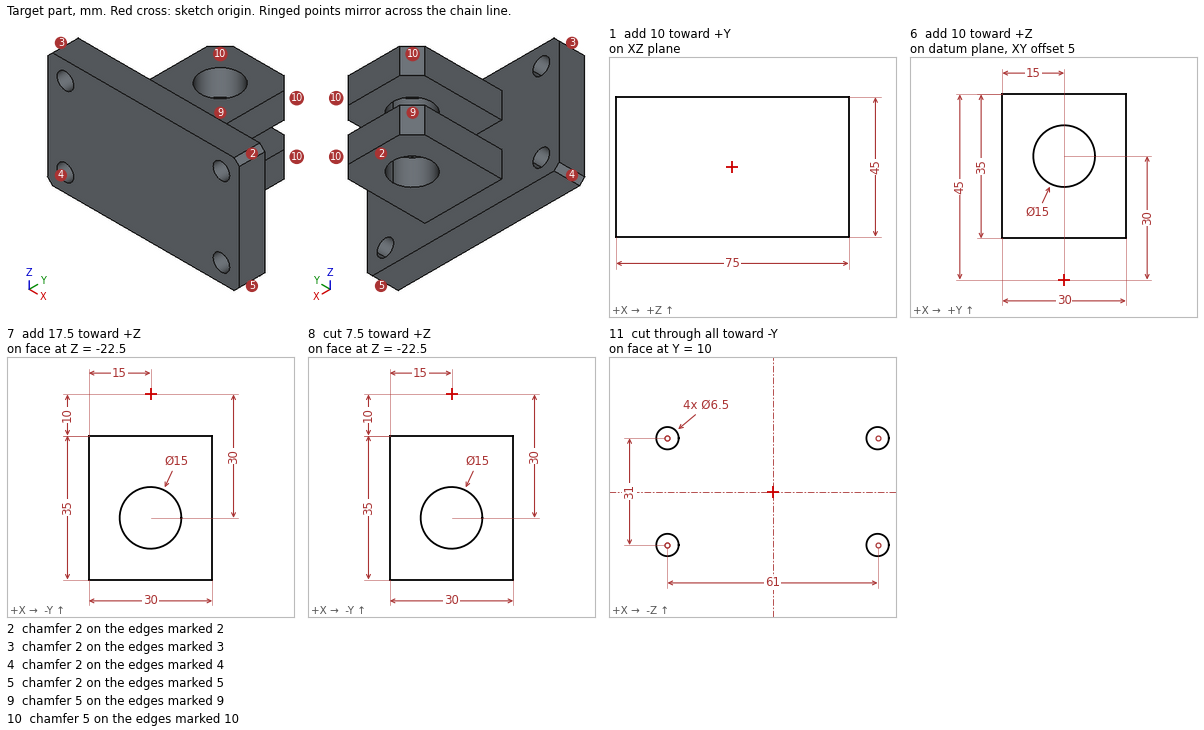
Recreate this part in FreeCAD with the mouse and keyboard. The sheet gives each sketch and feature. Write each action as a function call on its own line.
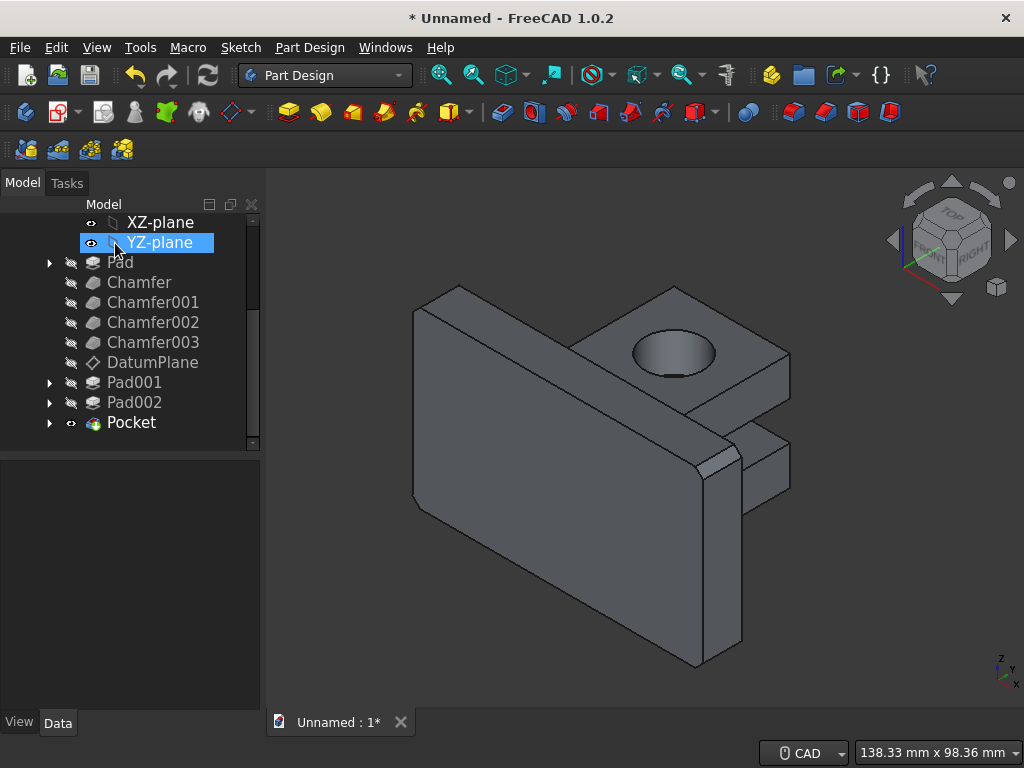
key(2)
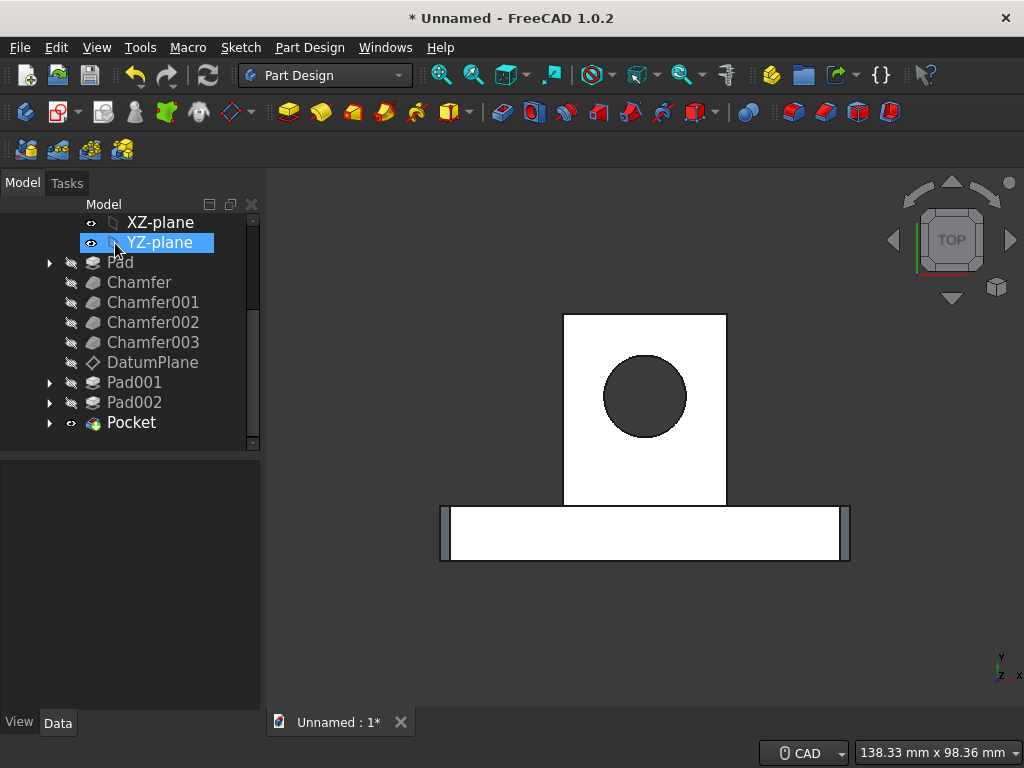
key(1)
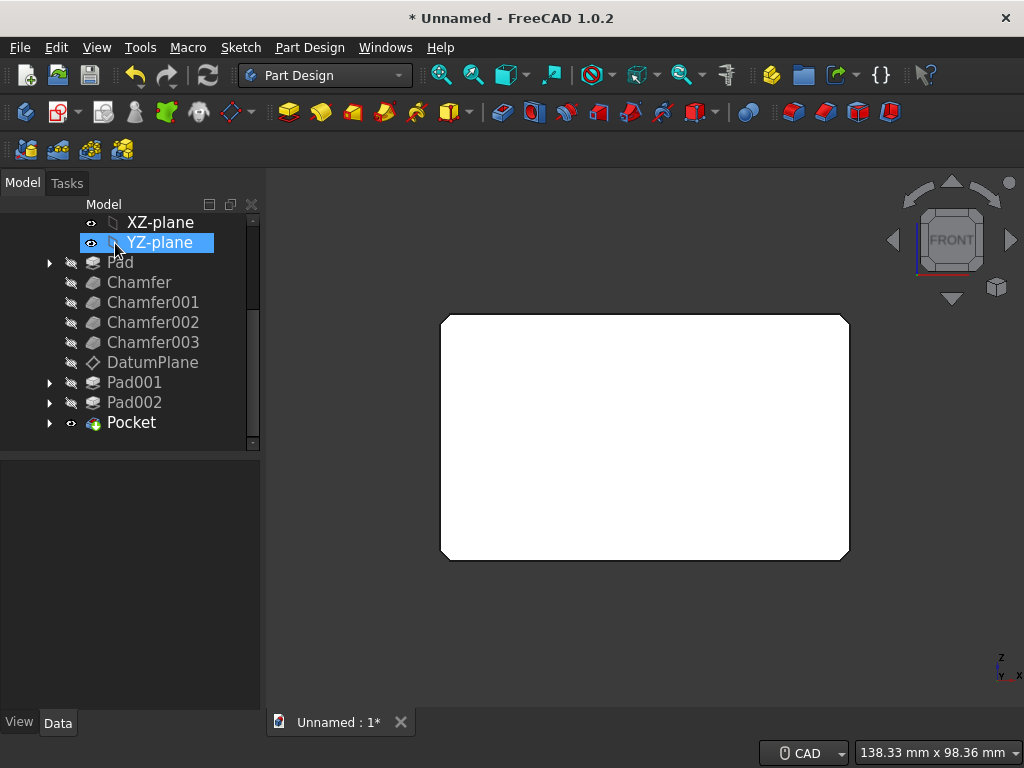
key(3)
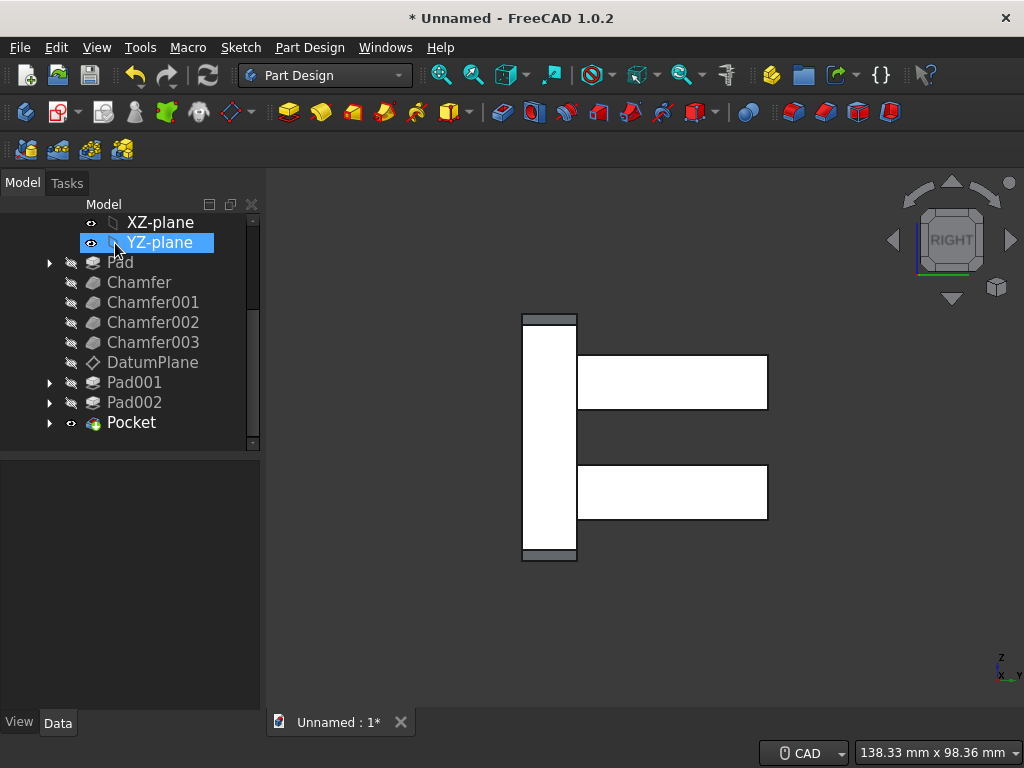
key(5)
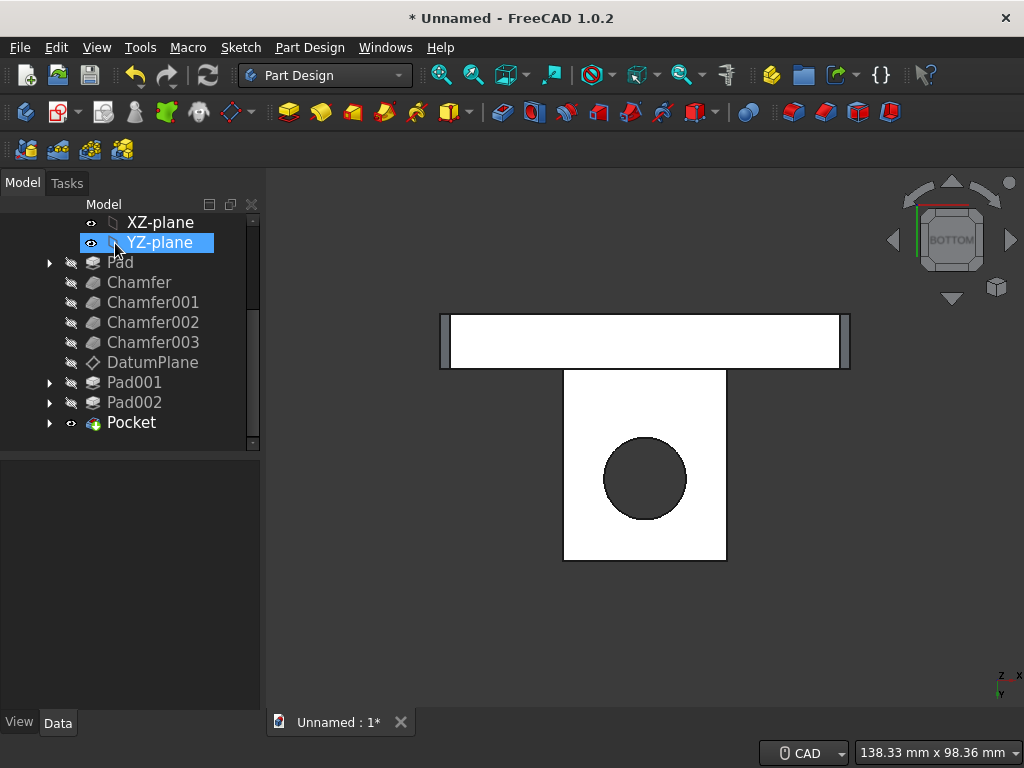
key(4)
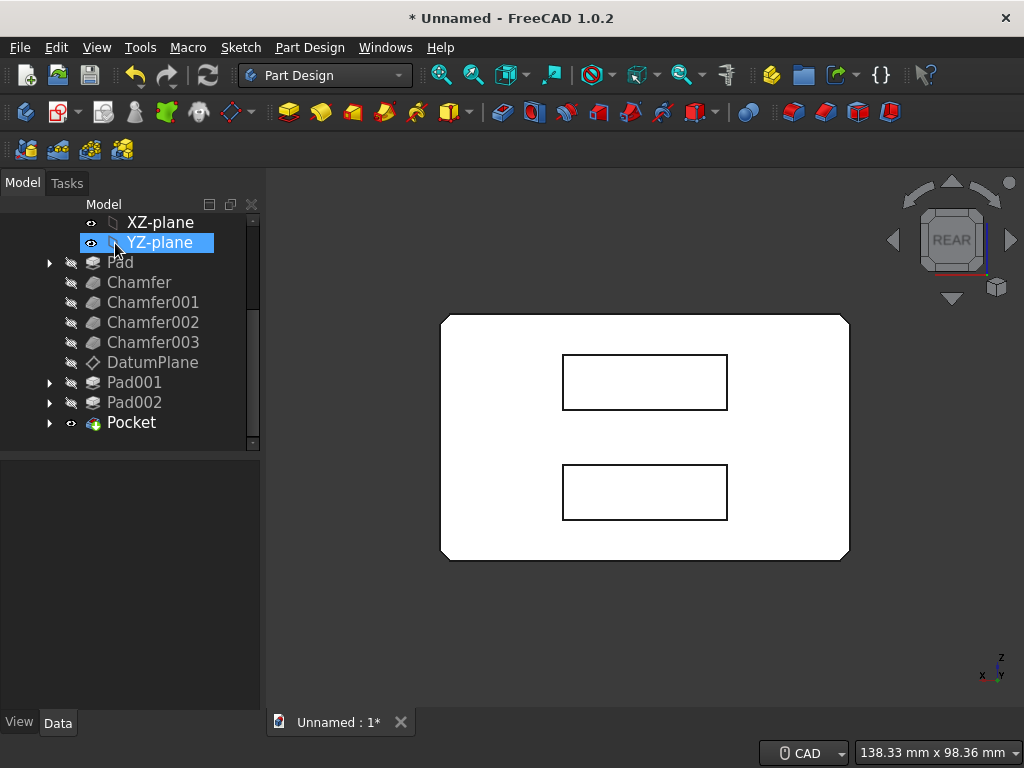
click(727, 491)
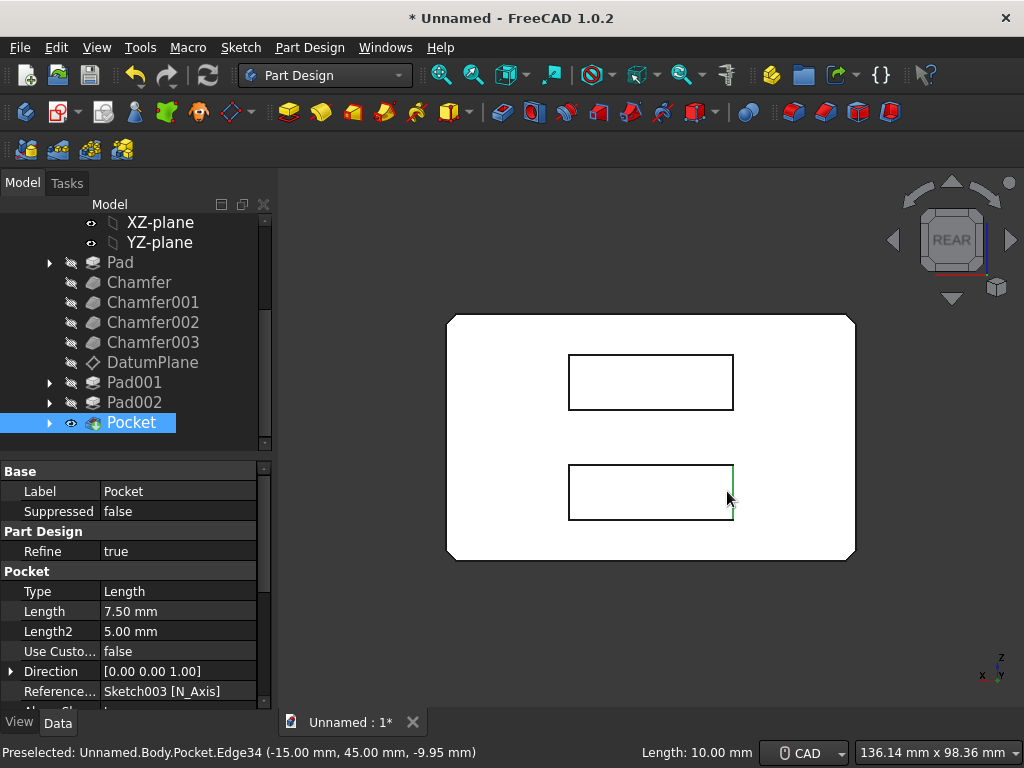
click(826, 112)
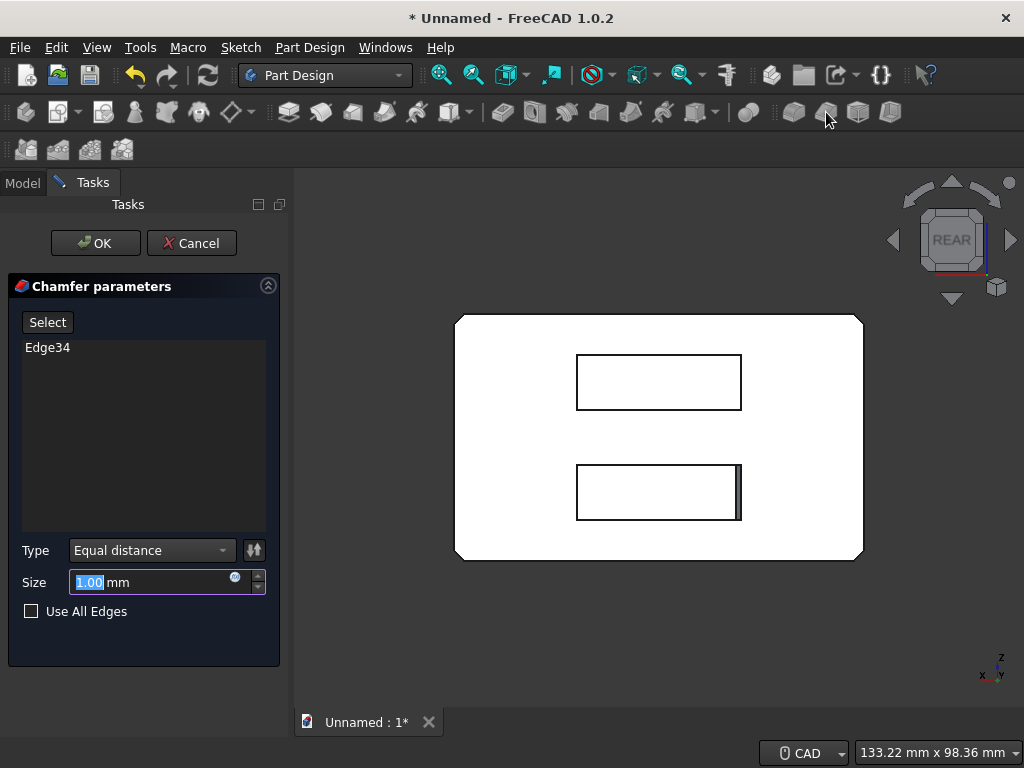
text(5)
key(Tab)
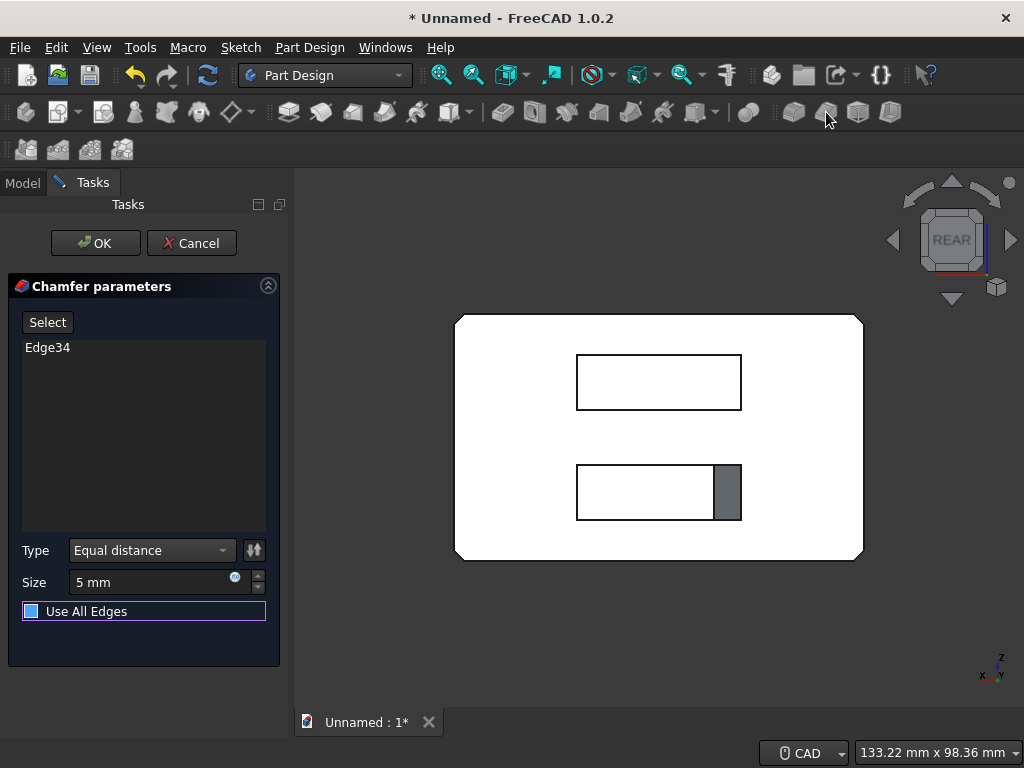
click(96, 243)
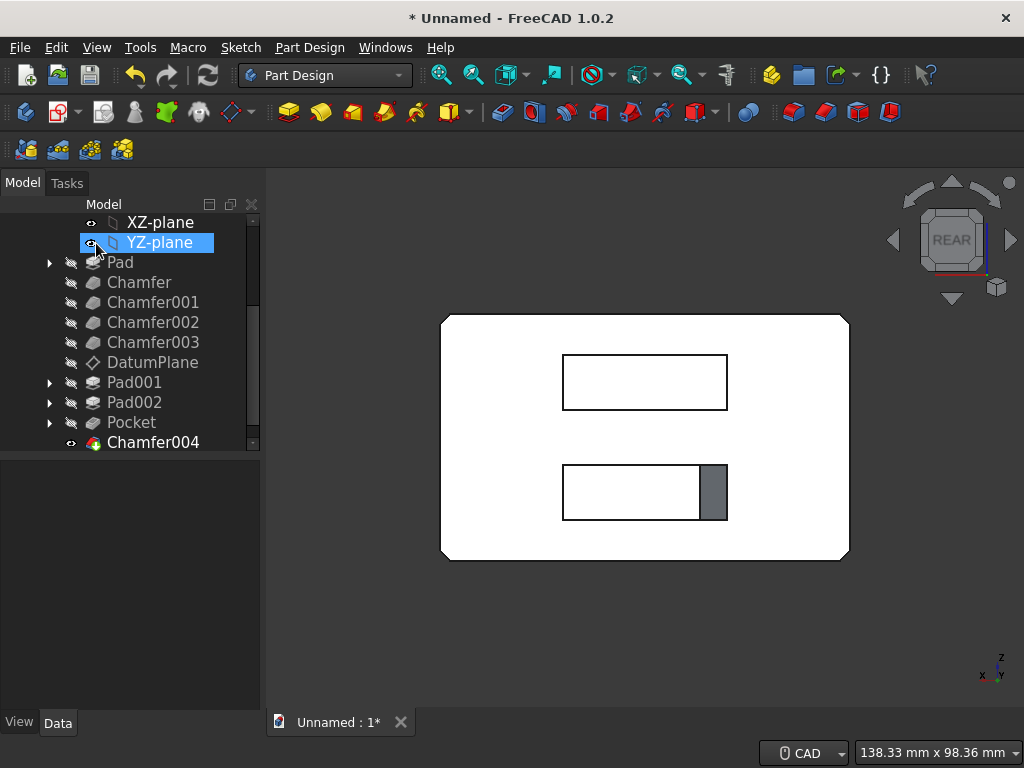
click(563, 382)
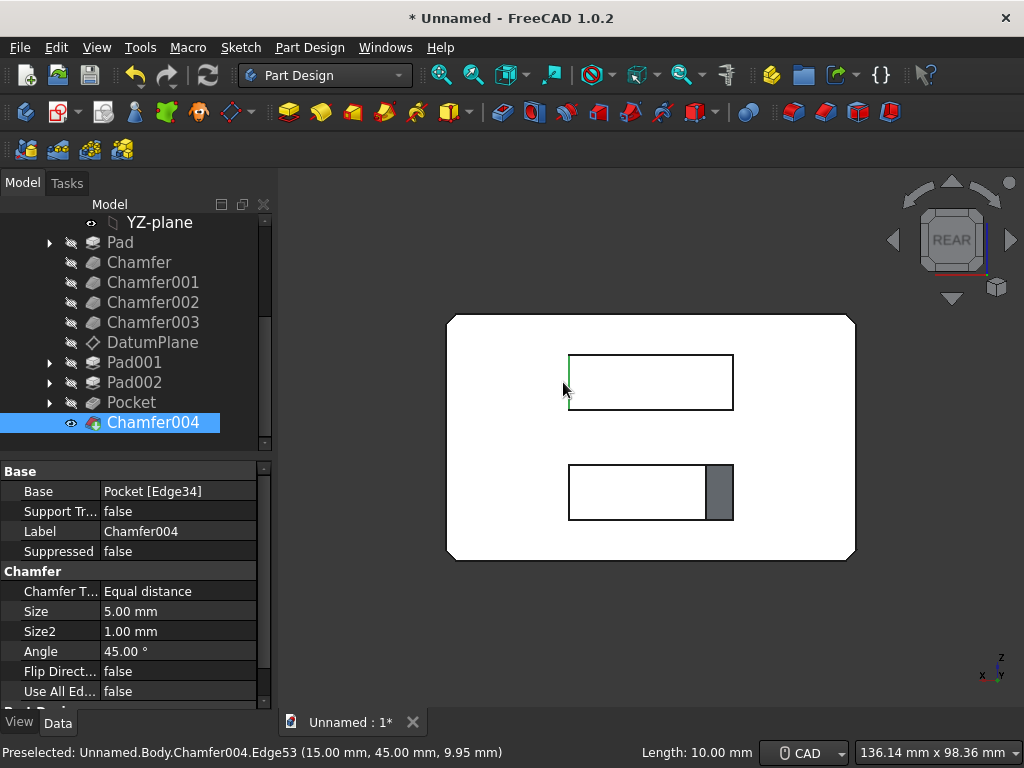
click(733, 382, ctrl)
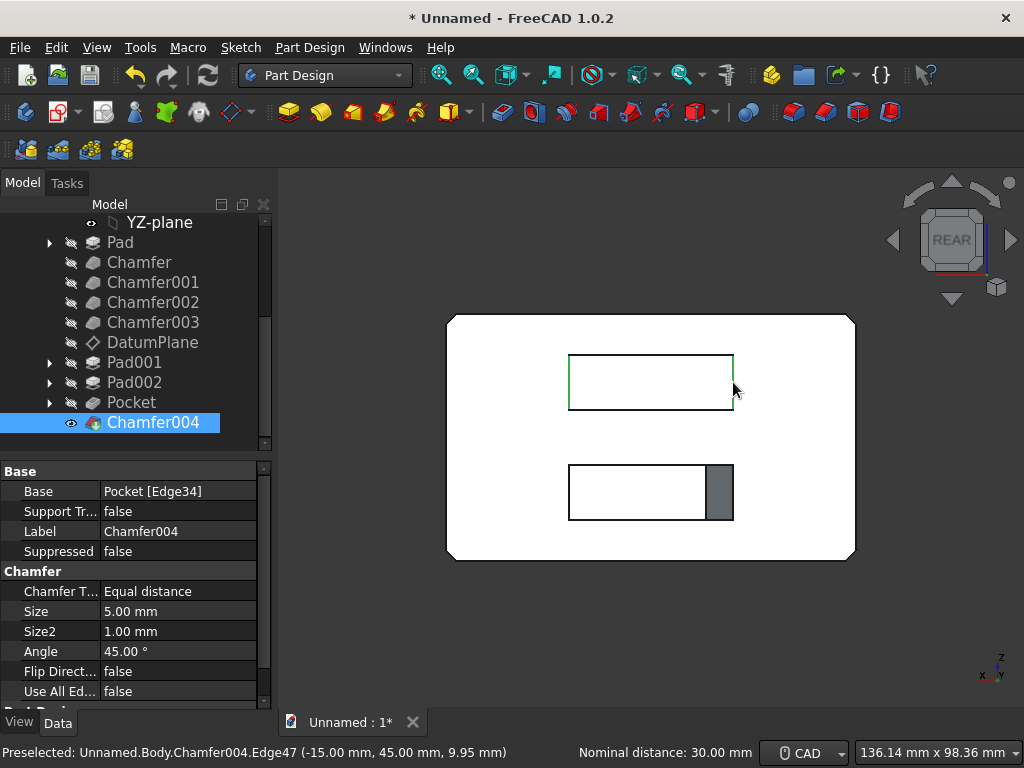
click(569, 491, ctrl)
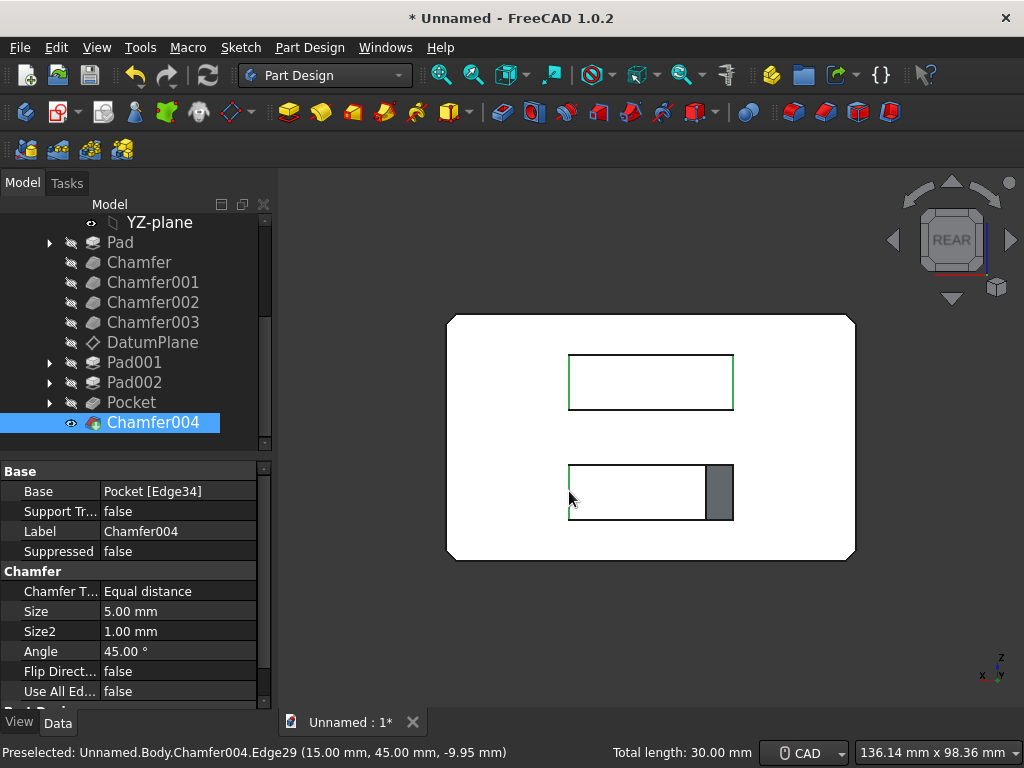
click(826, 112)